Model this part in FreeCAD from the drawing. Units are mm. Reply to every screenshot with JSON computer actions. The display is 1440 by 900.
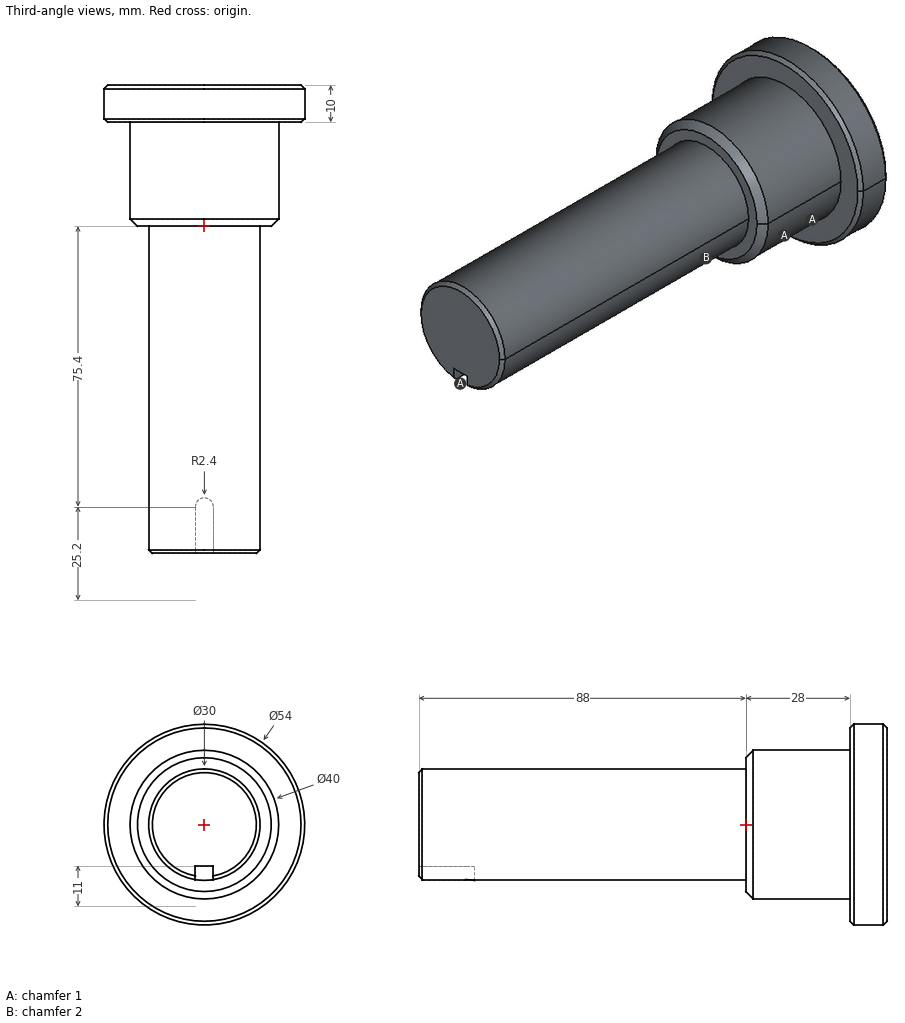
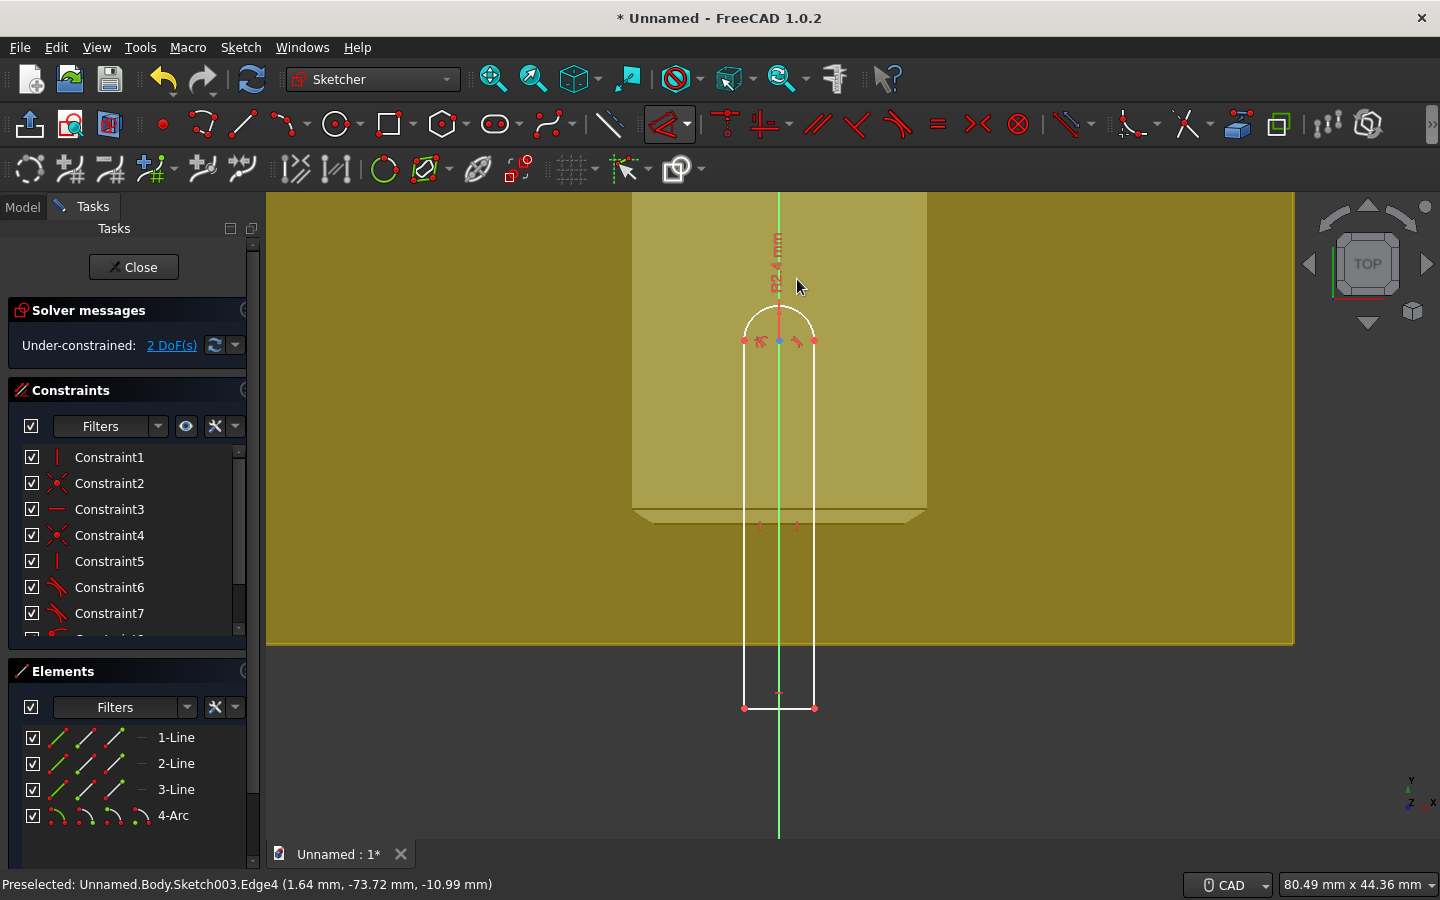
{"action": "left_click", "coordinate": [744, 451]}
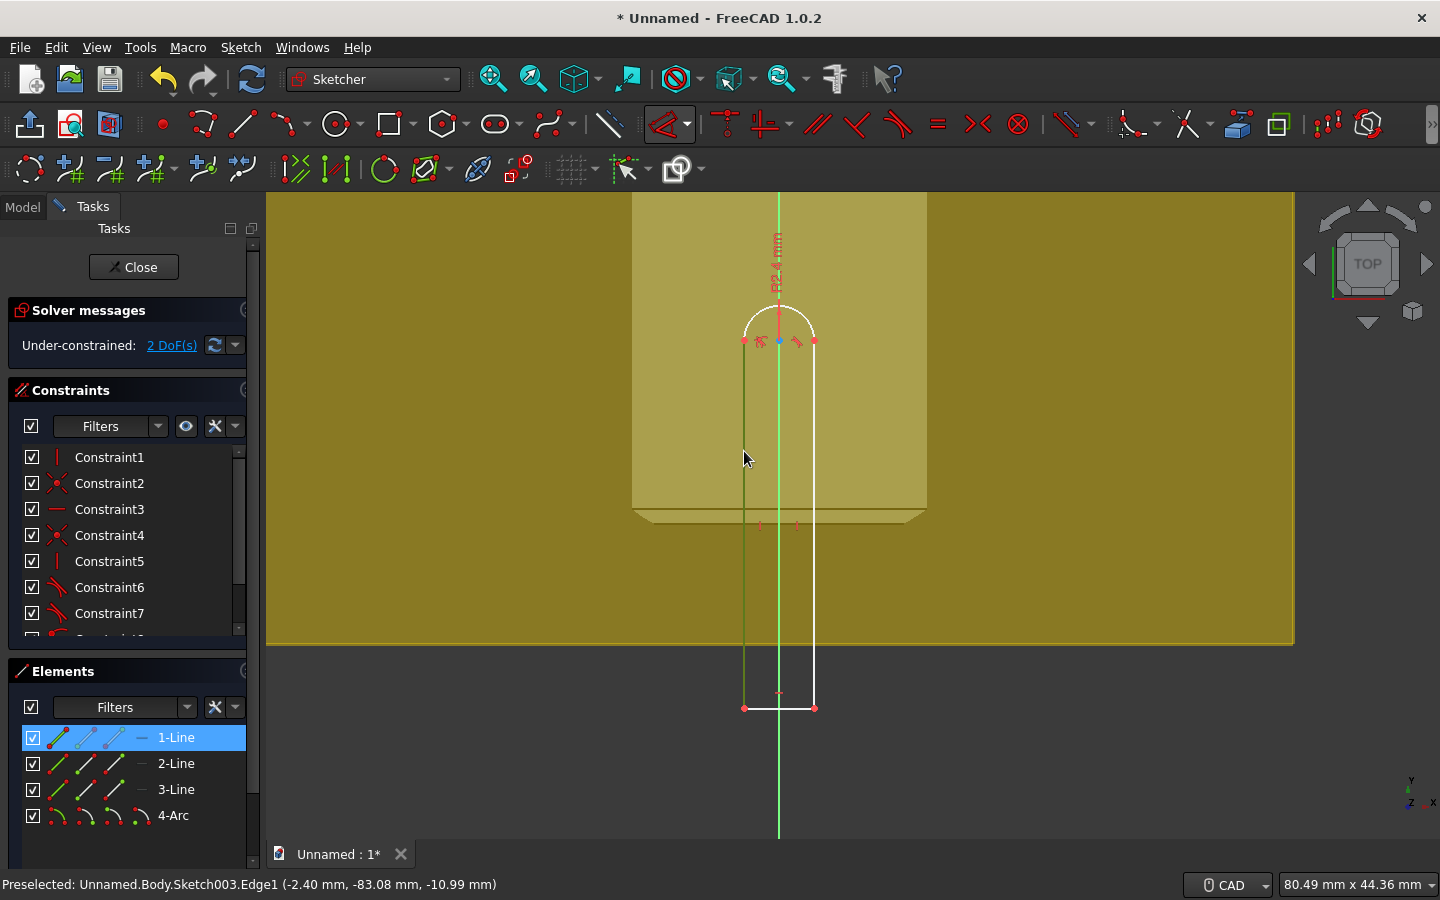
{"action": "key", "text": "i"}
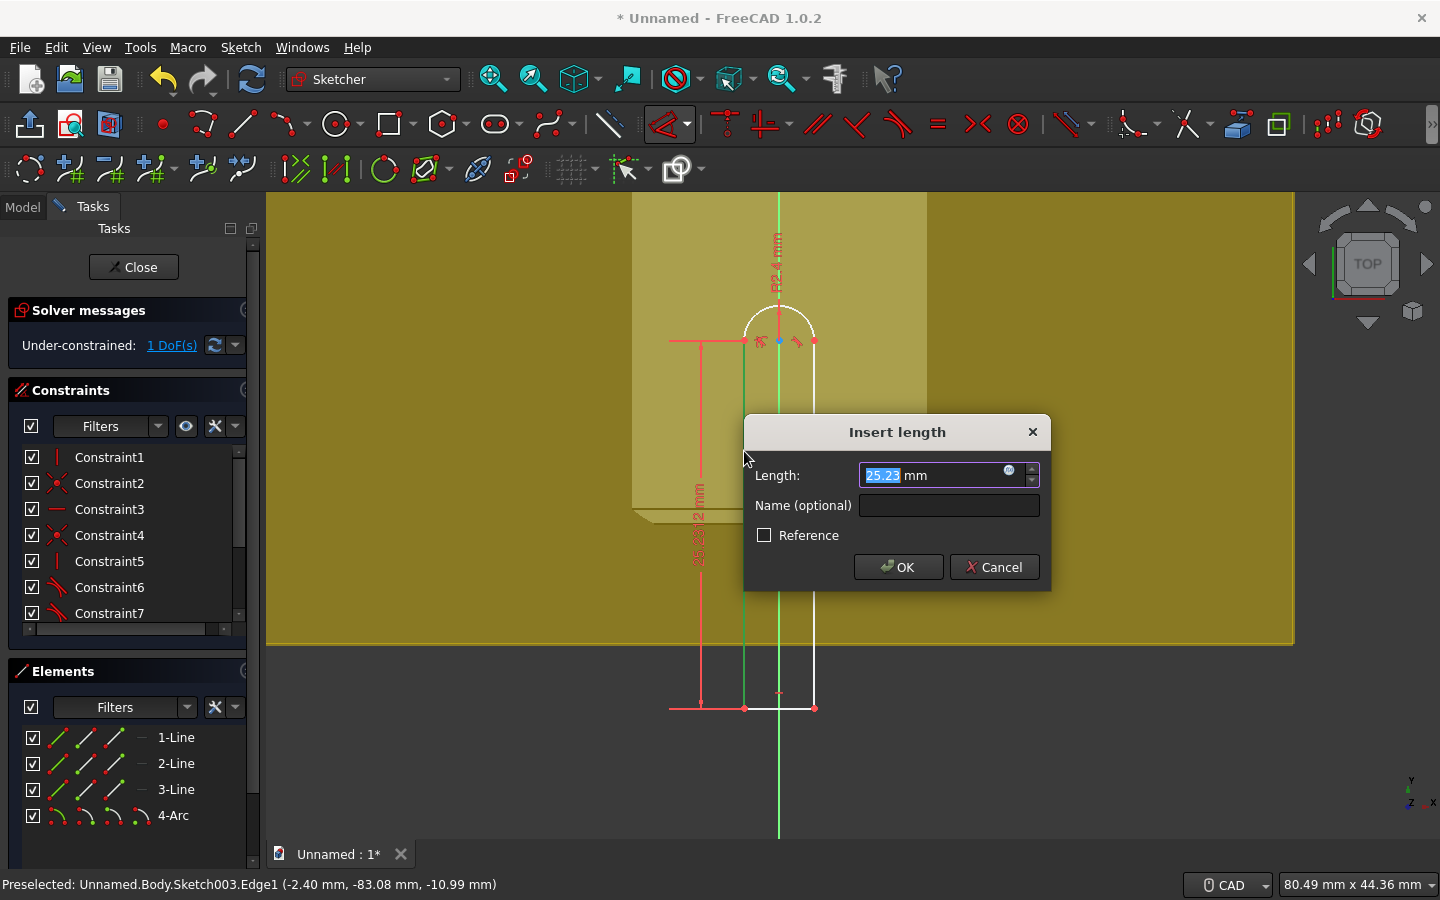
{"action": "type", "text": "25.2"}
{"action": "key", "text": "Return"}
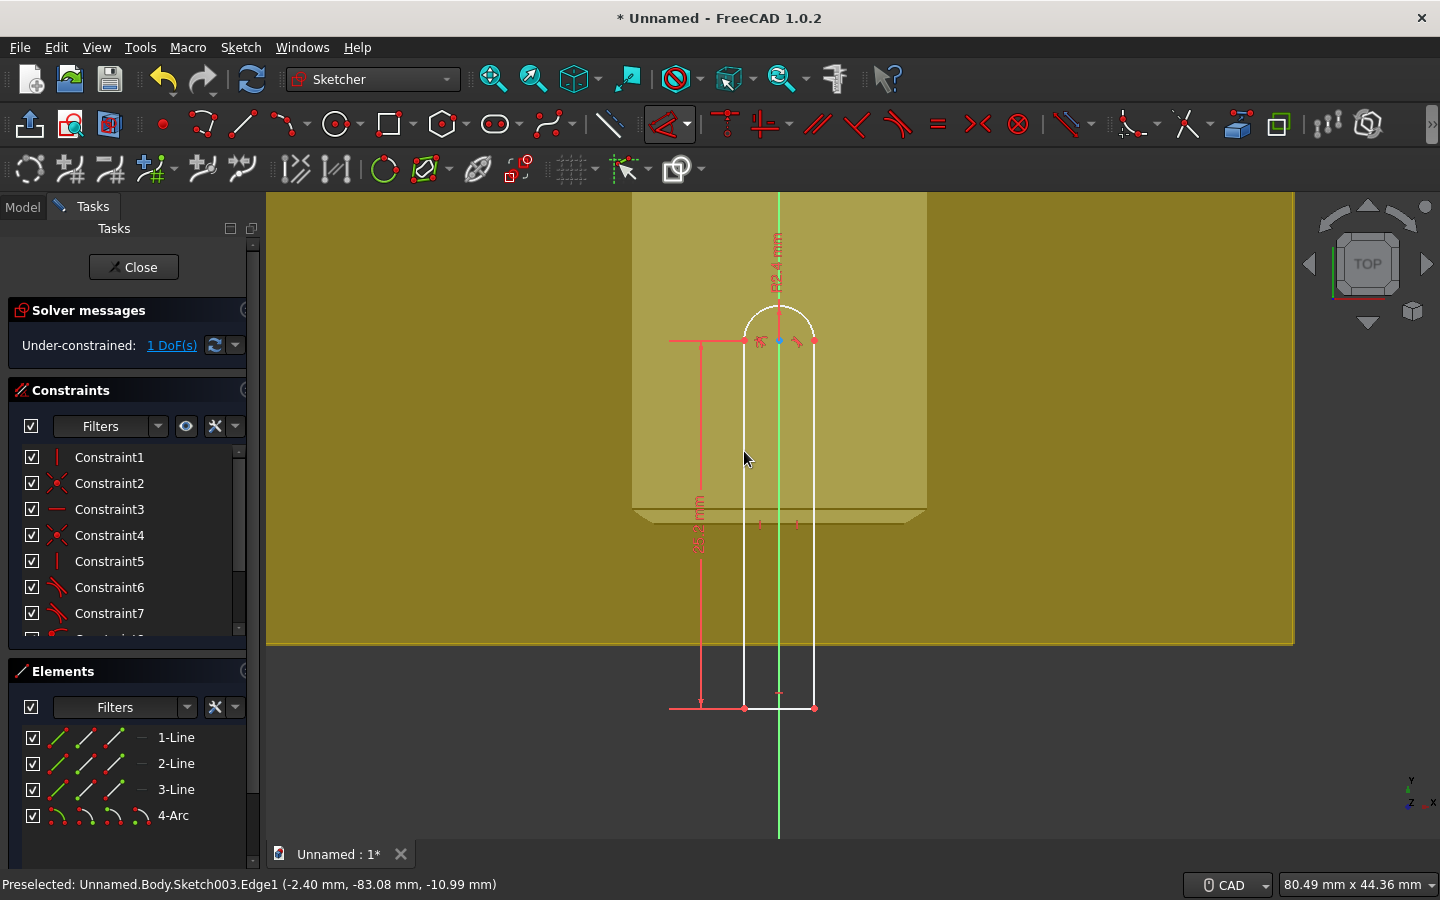
{"action": "left_click", "coordinate": [744, 341]}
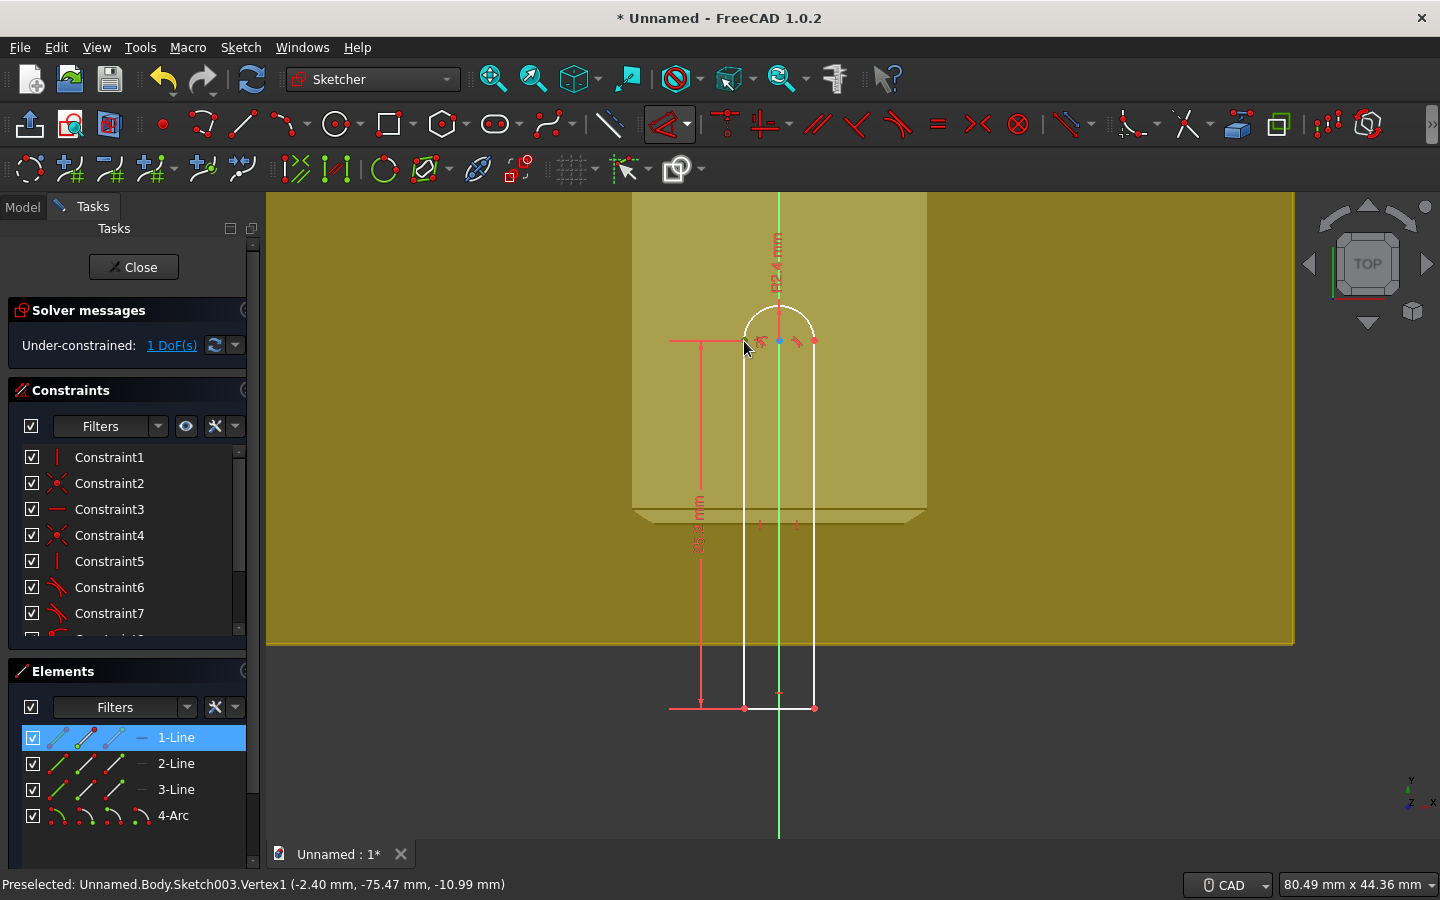
{"action": "key", "text": "i"}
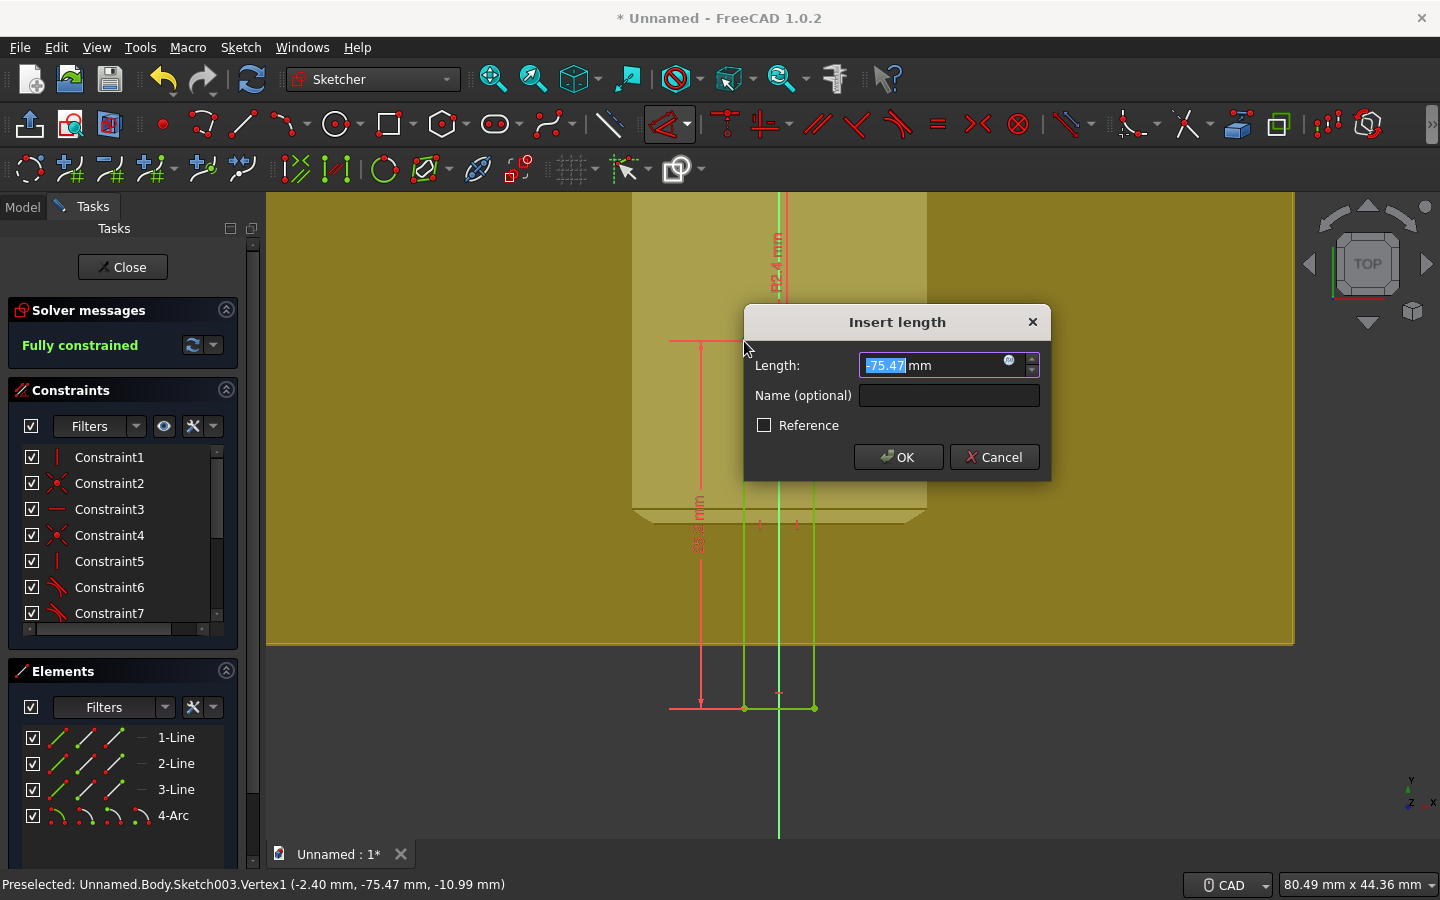
{"action": "type", "text": "-75.4"}
{"action": "key", "text": "Return"}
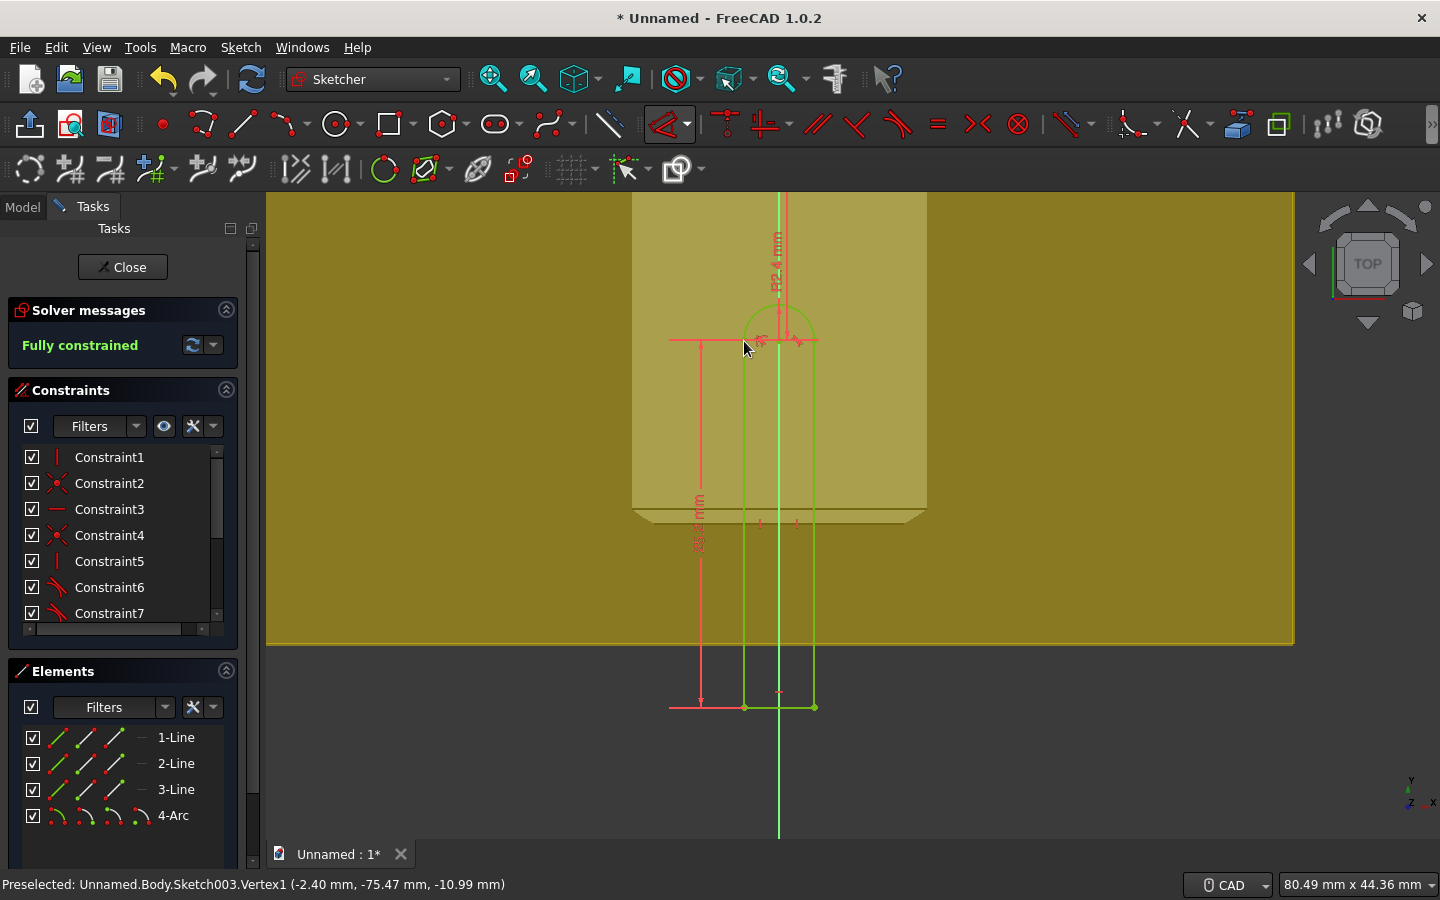
{"action": "left_click", "coordinate": [123, 267]}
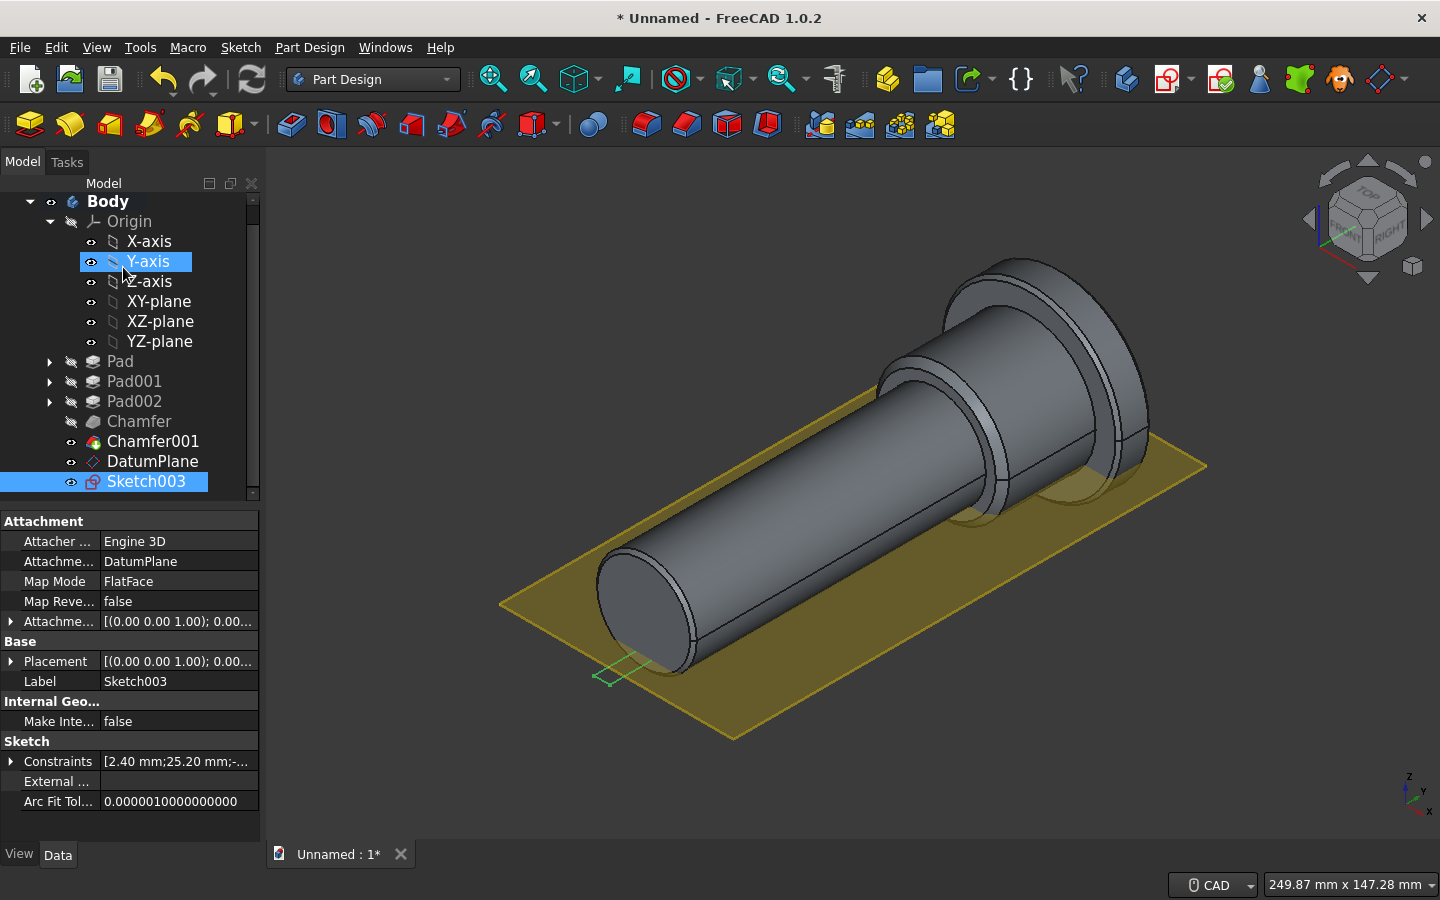
{"action": "left_click", "coordinate": [292, 124]}